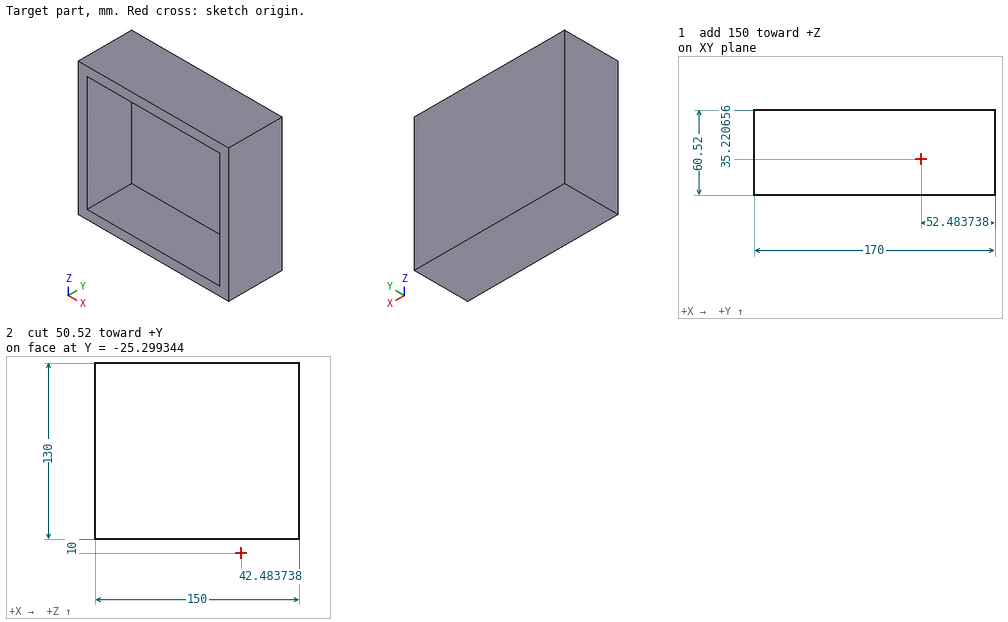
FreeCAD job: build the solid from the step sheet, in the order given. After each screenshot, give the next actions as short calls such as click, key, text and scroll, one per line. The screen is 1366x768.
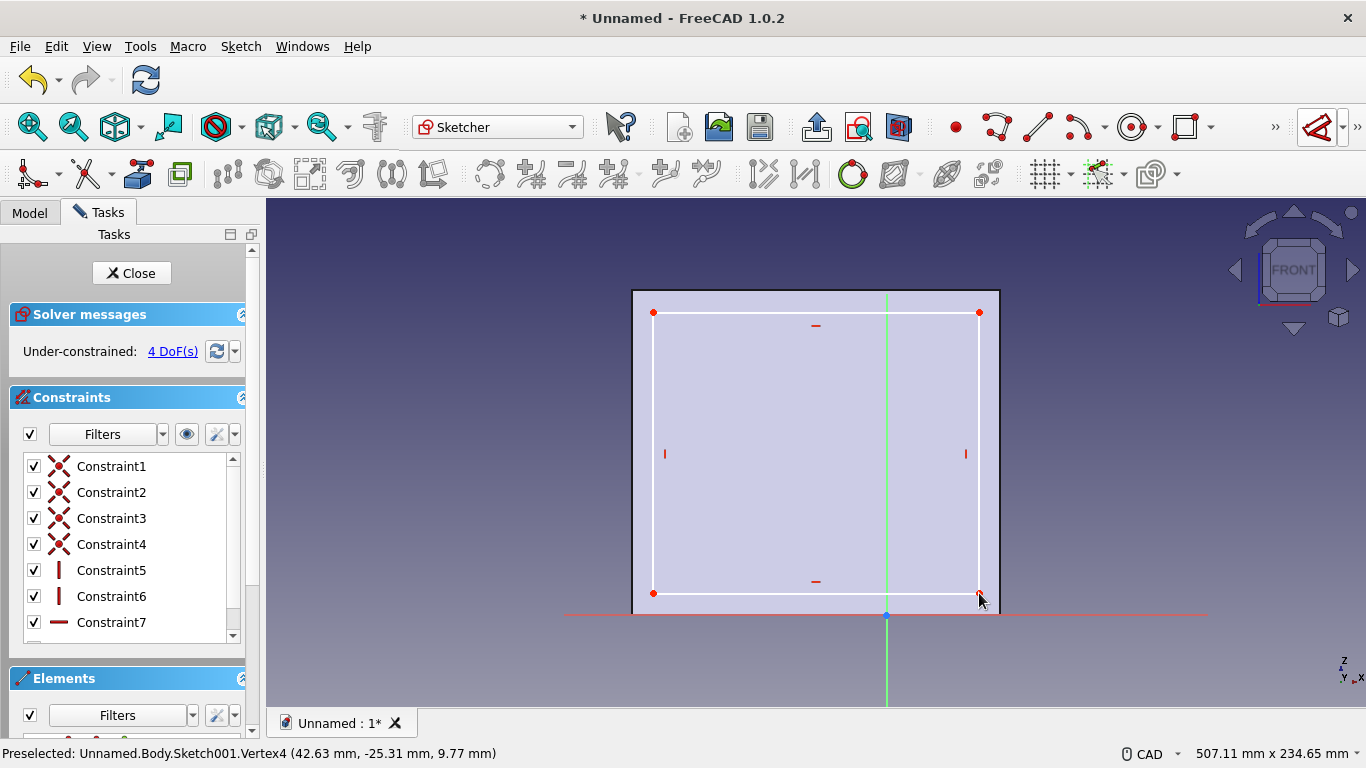
click(653, 397)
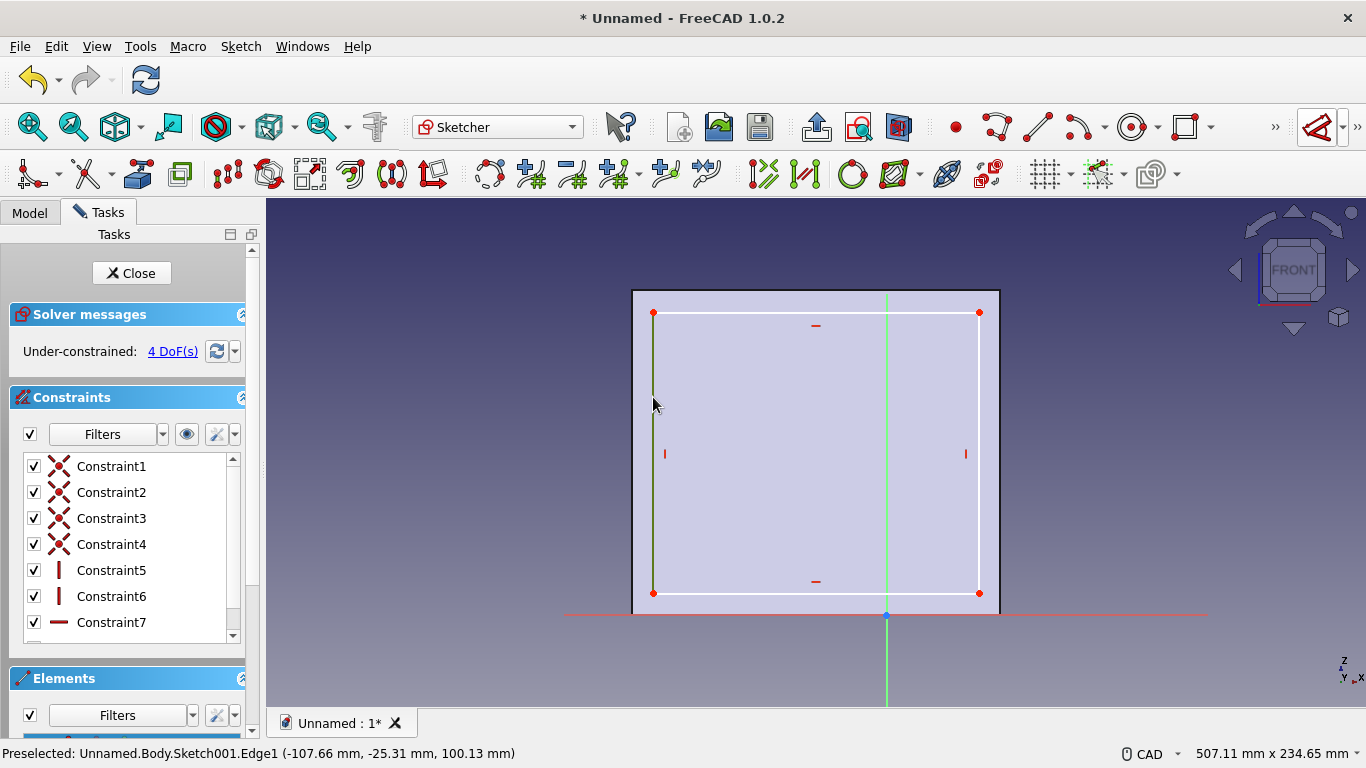
key(i)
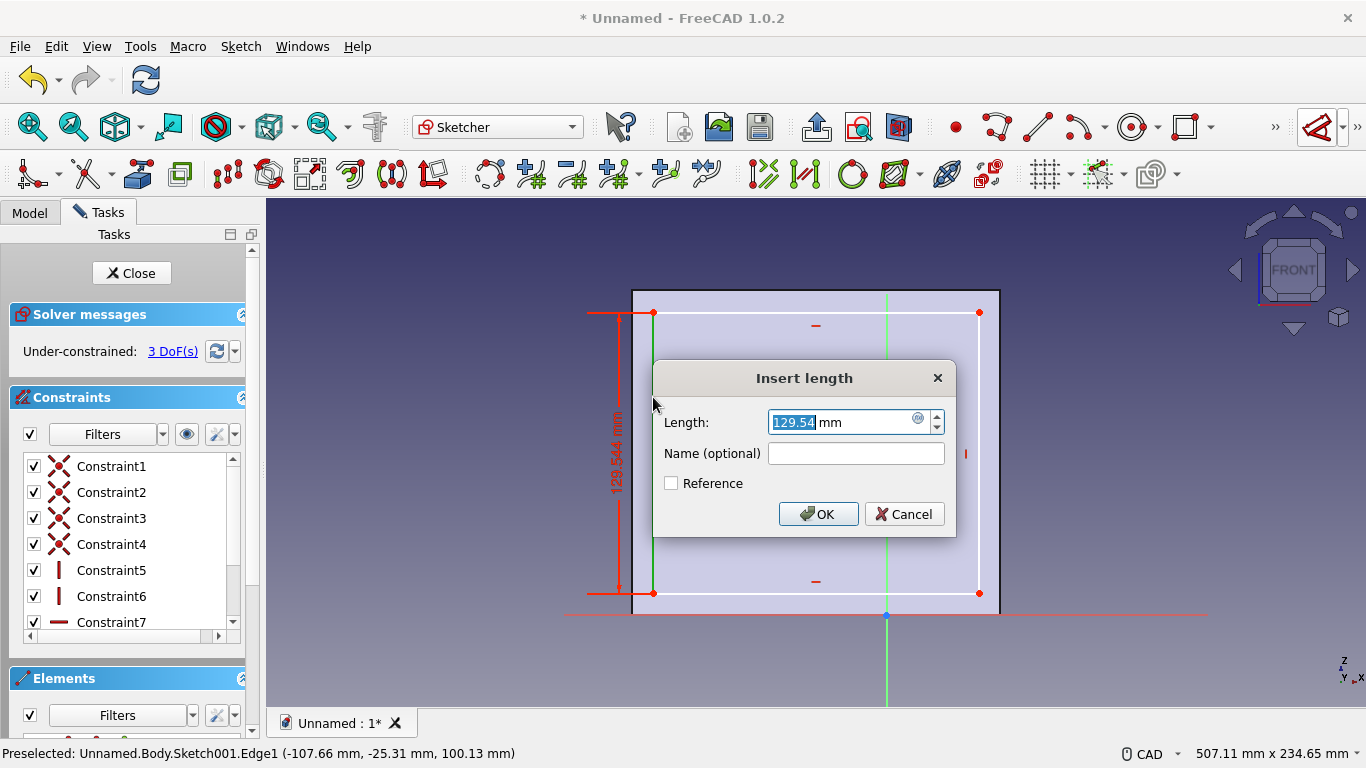
text(130)
key(Return)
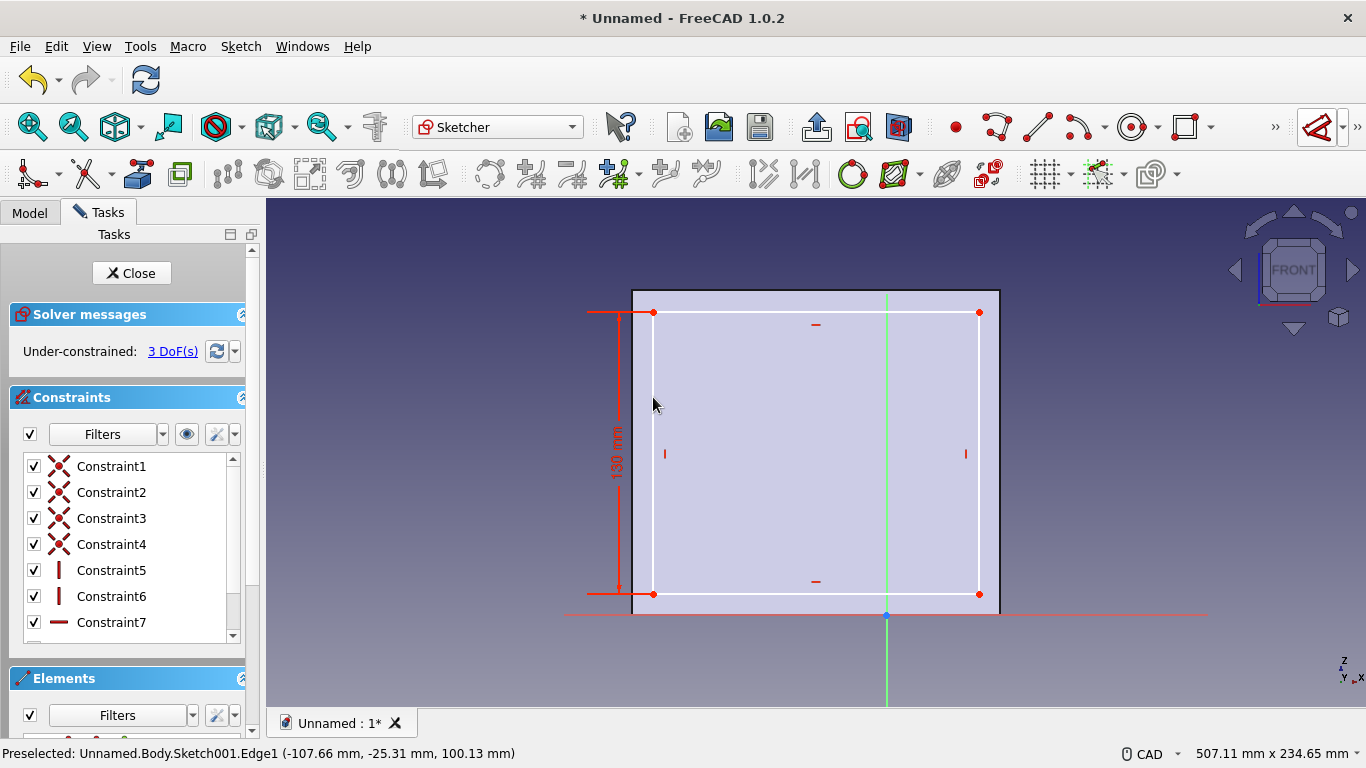
click(751, 594)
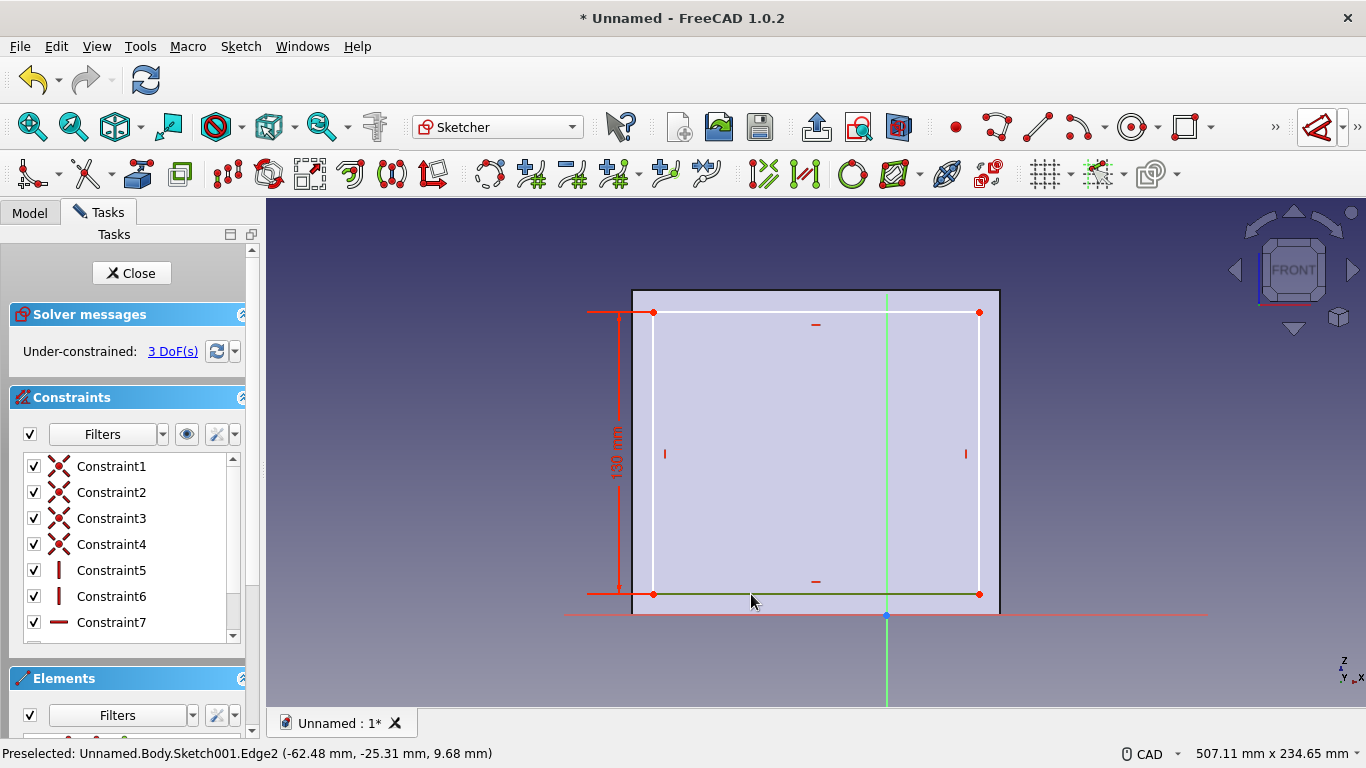
click(1342, 128)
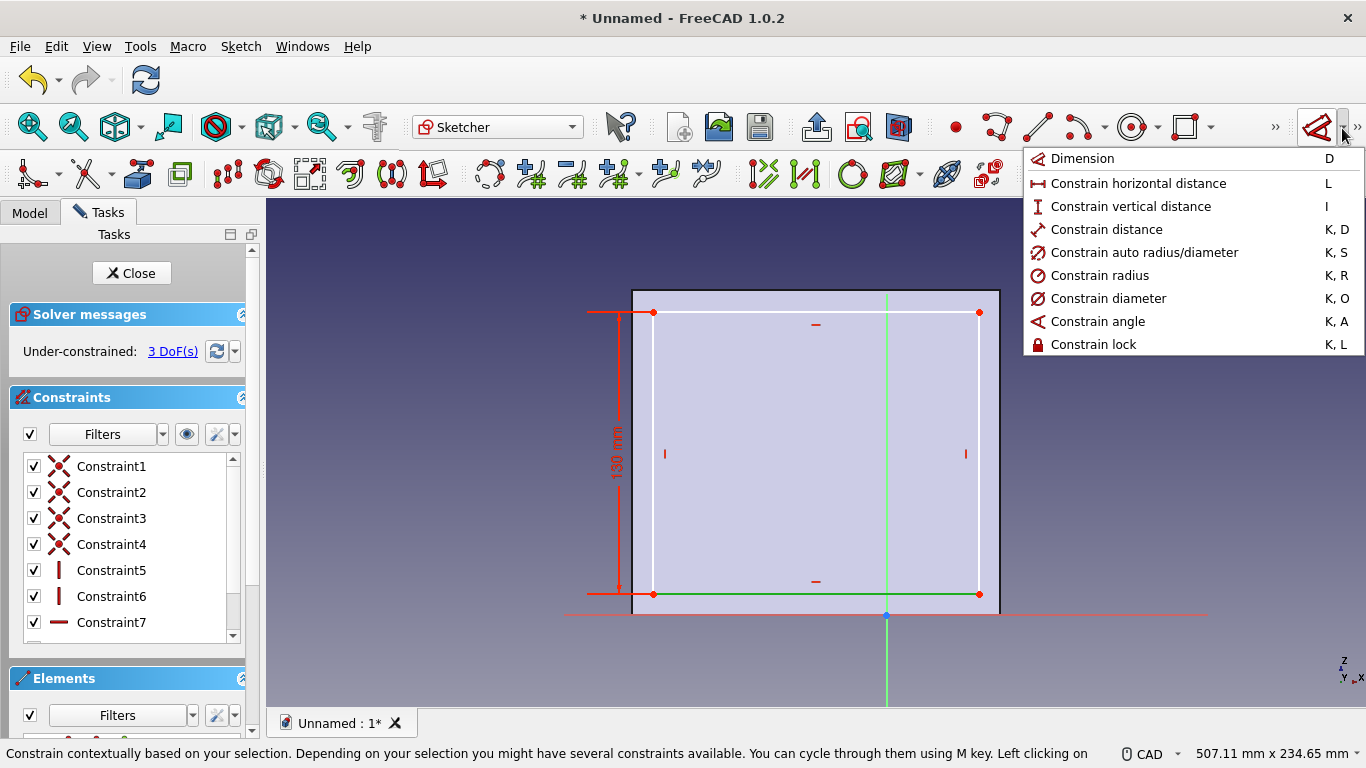
click(1194, 184)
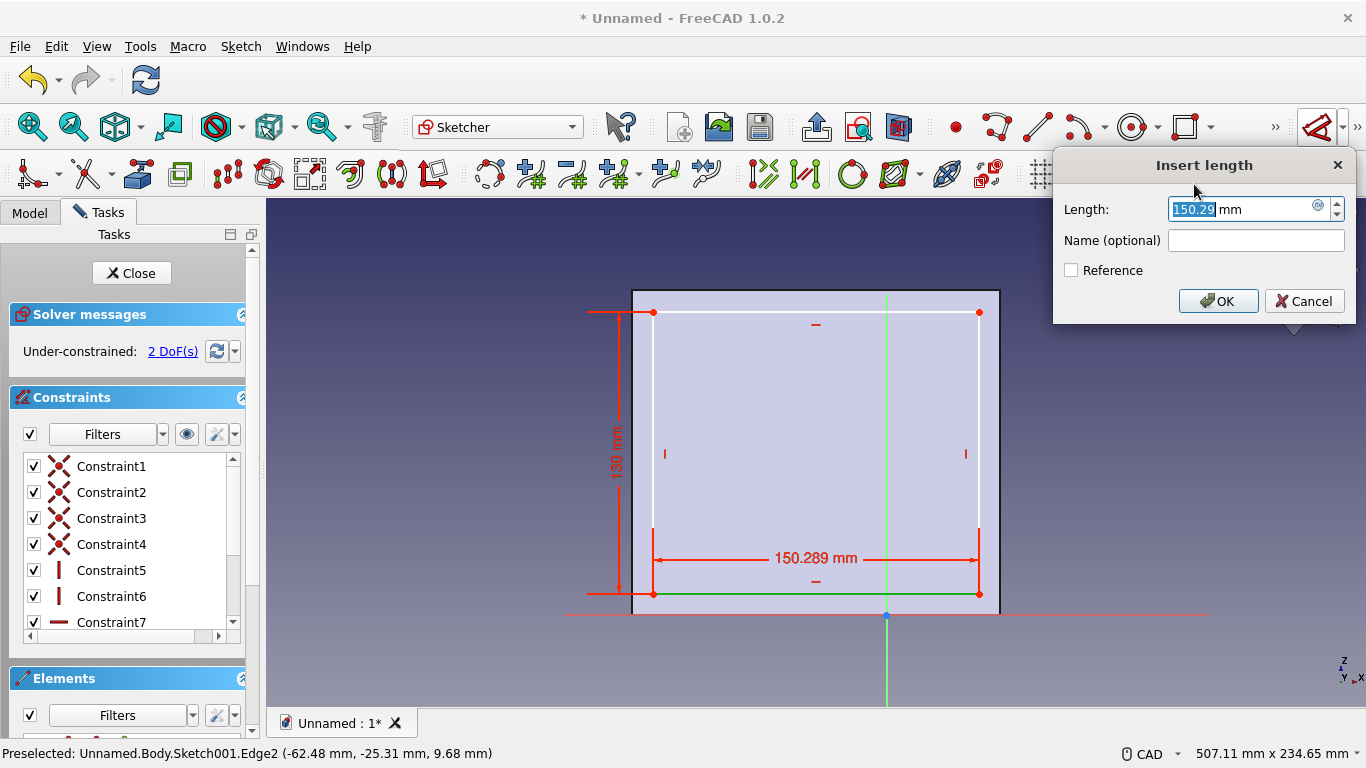
text(150)
key(Return)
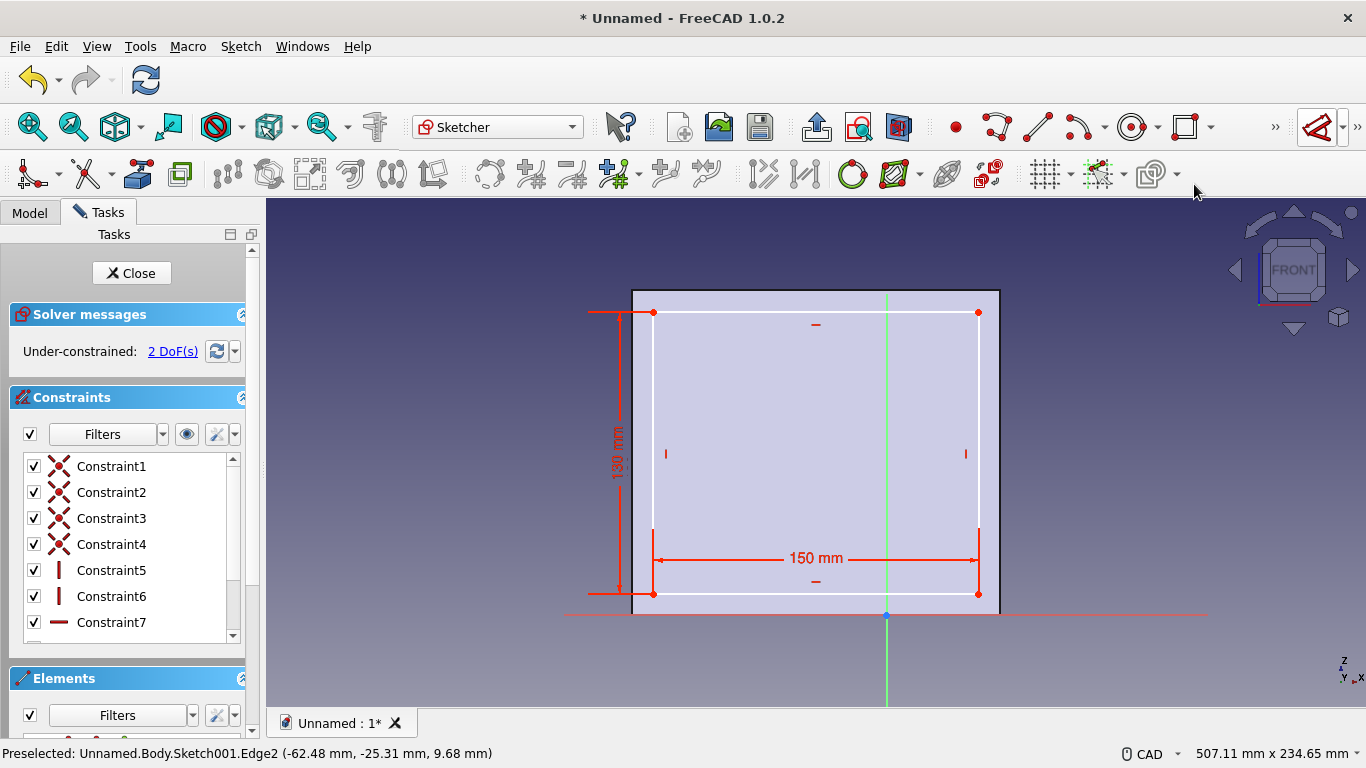
scroll(653, 594, up, 4)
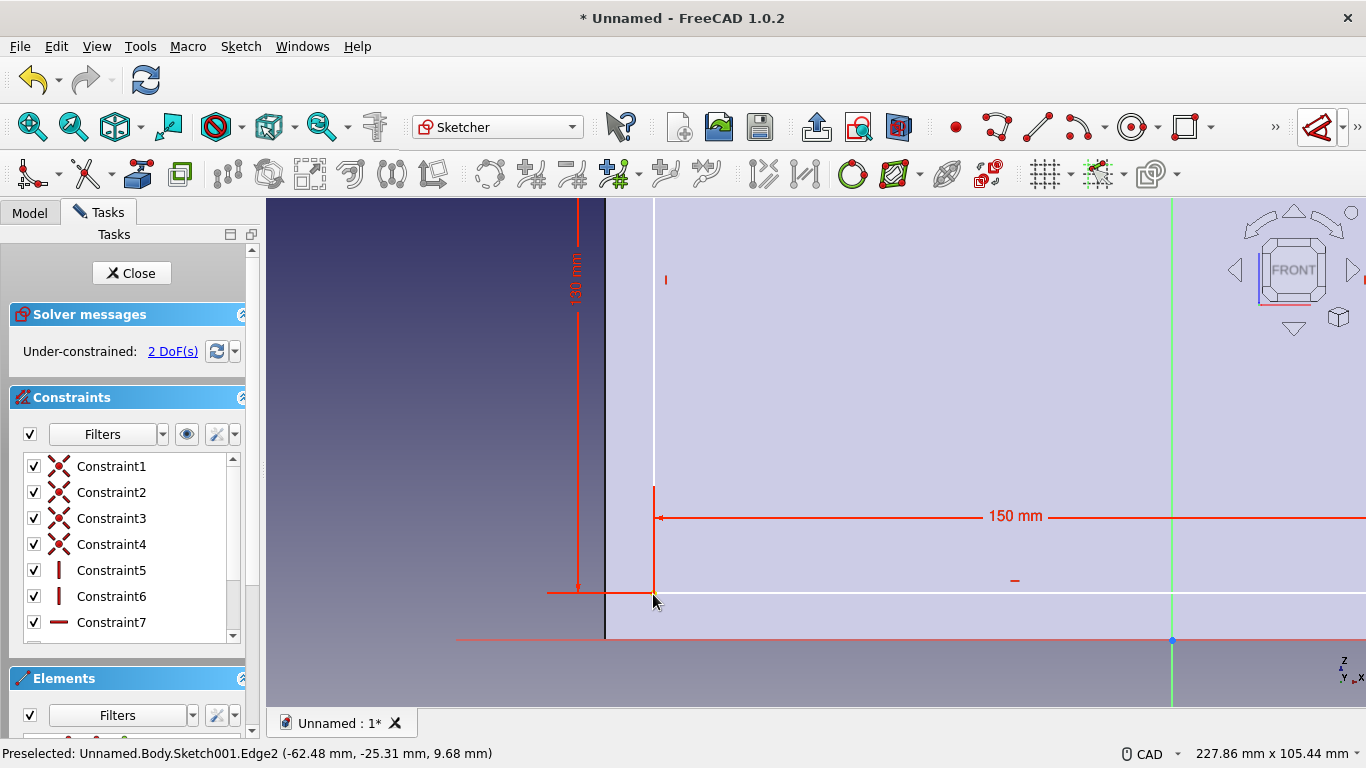
click(654, 593)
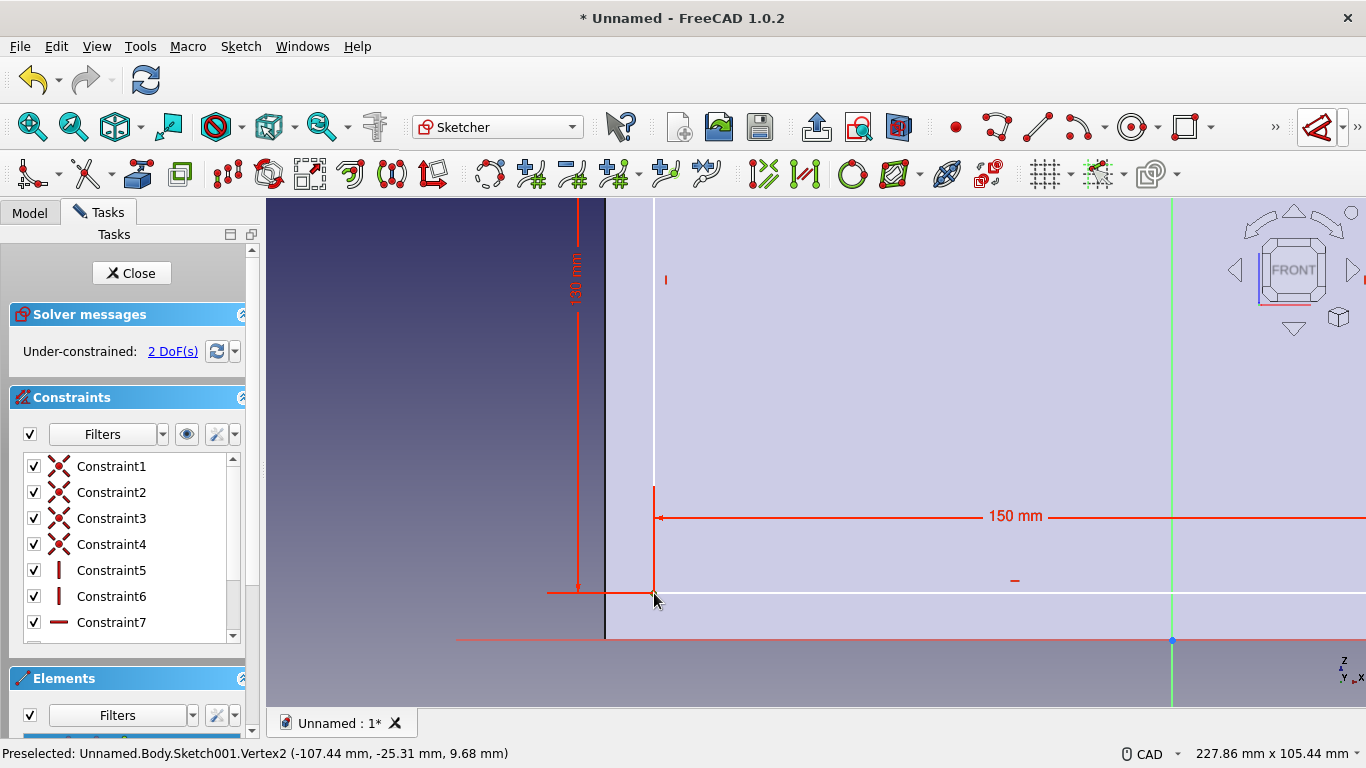
click(1342, 128)